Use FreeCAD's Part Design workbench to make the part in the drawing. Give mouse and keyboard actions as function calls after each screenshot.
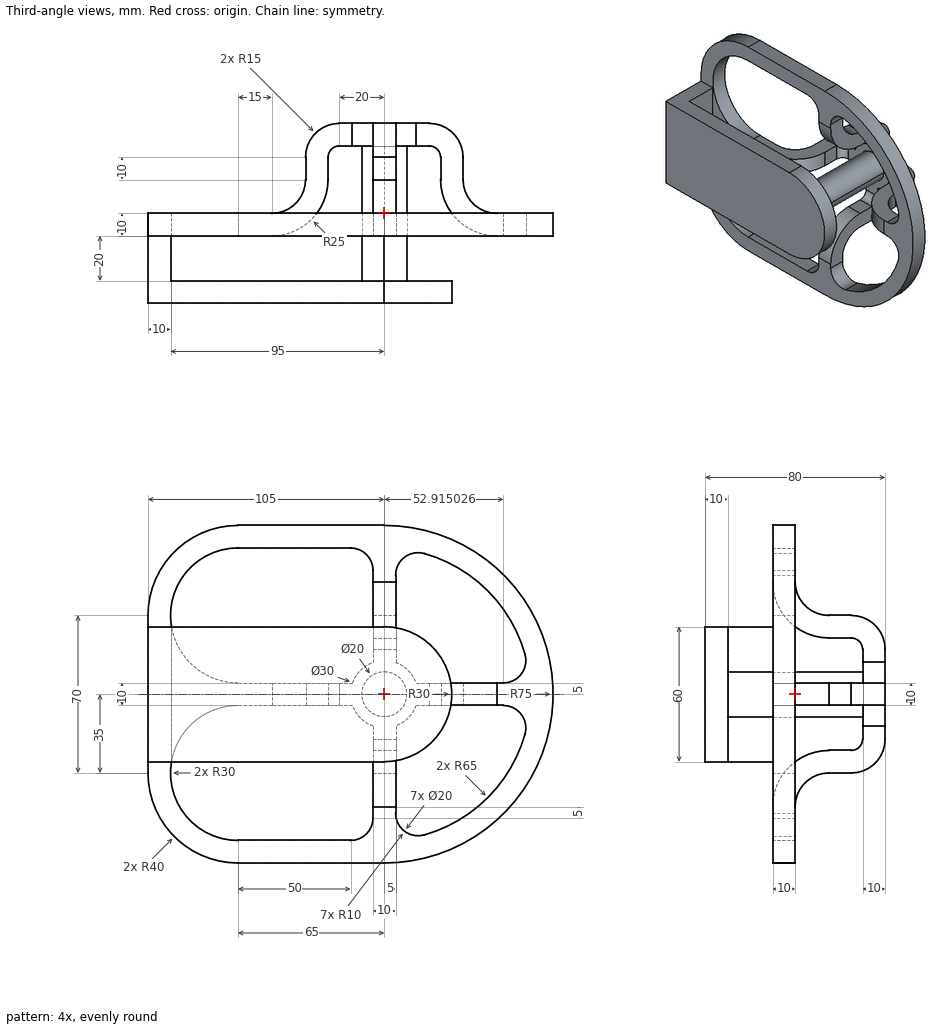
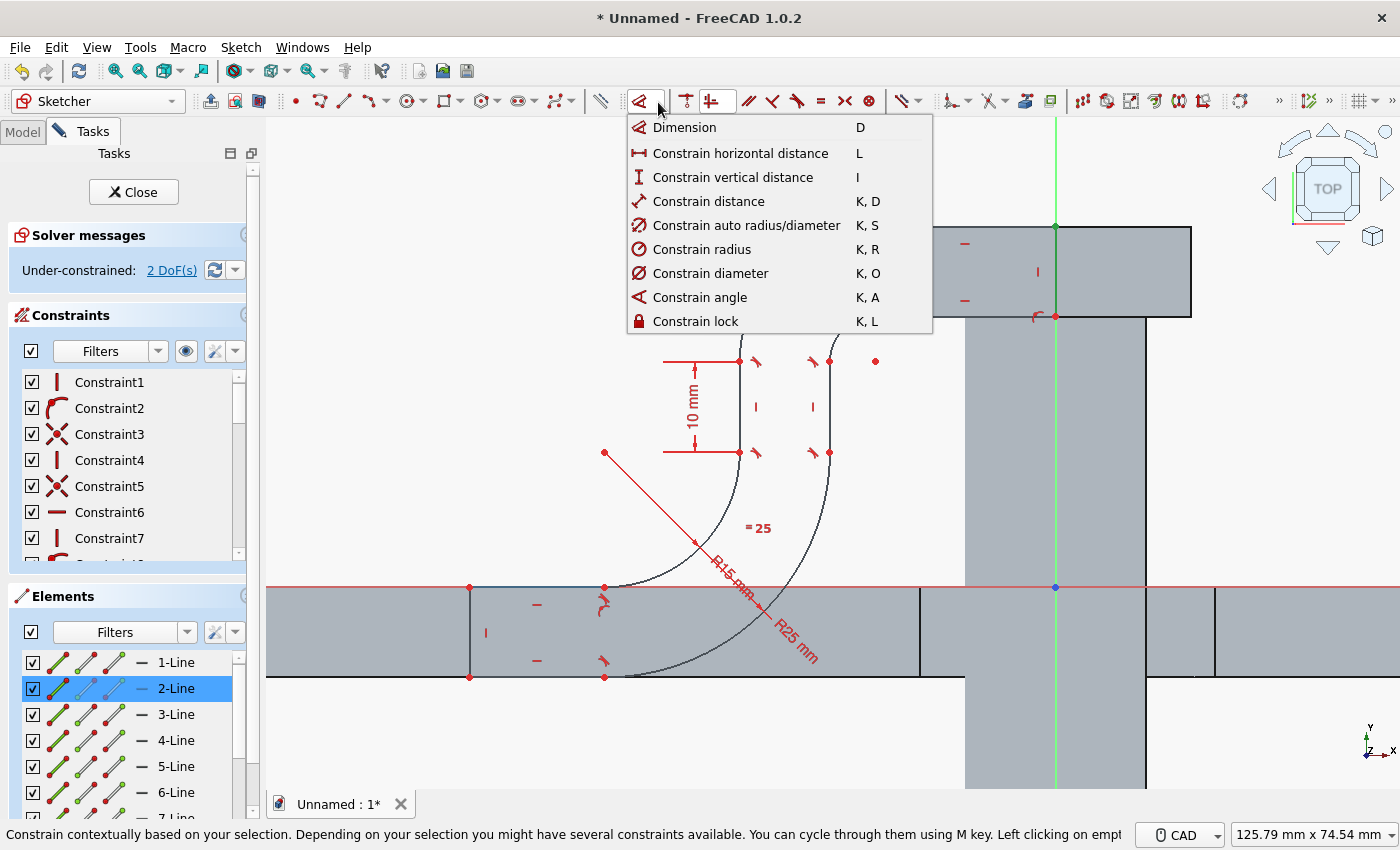
click(780, 153)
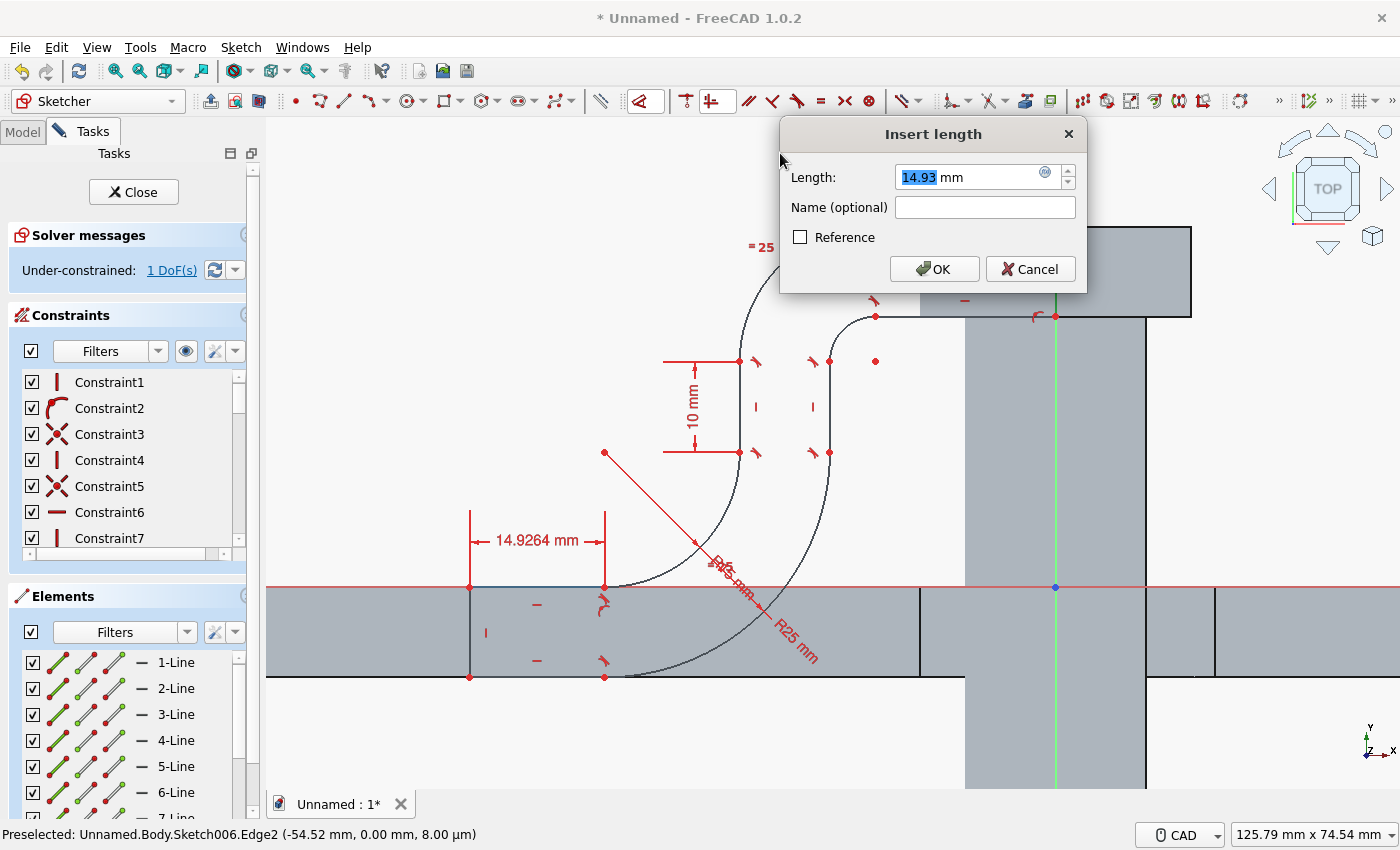
text(15)
key(Return)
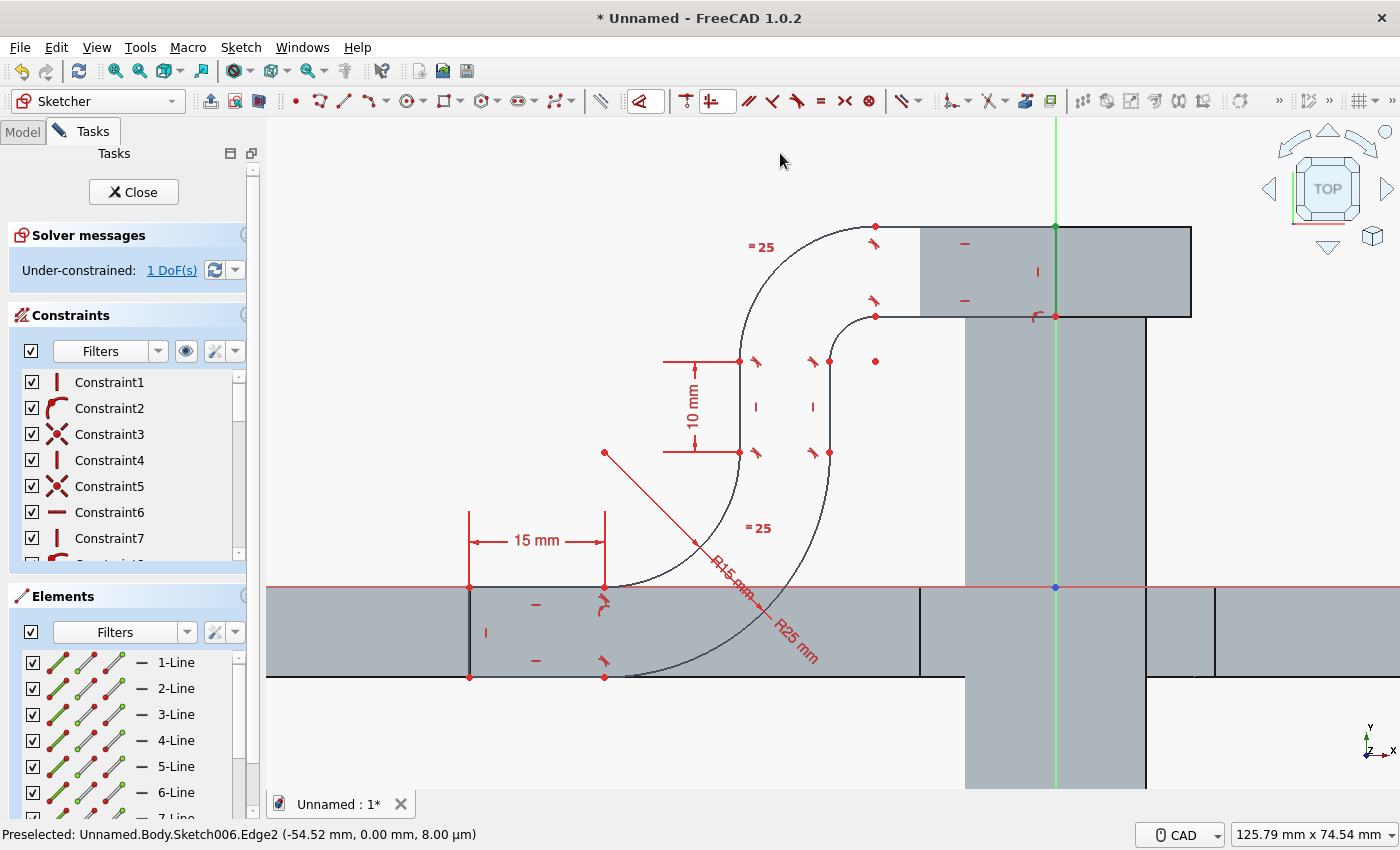
click(929, 317)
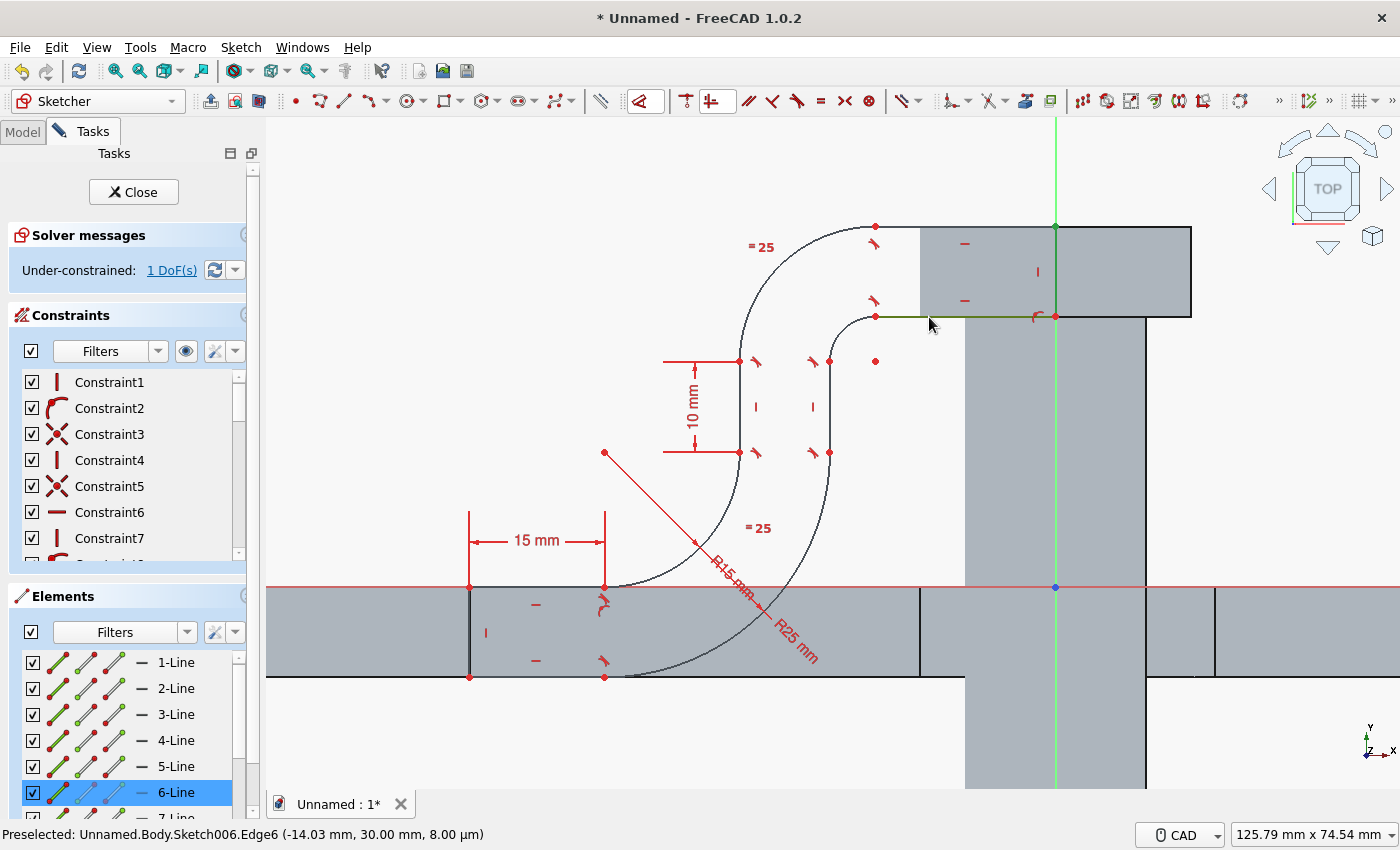
click(658, 102)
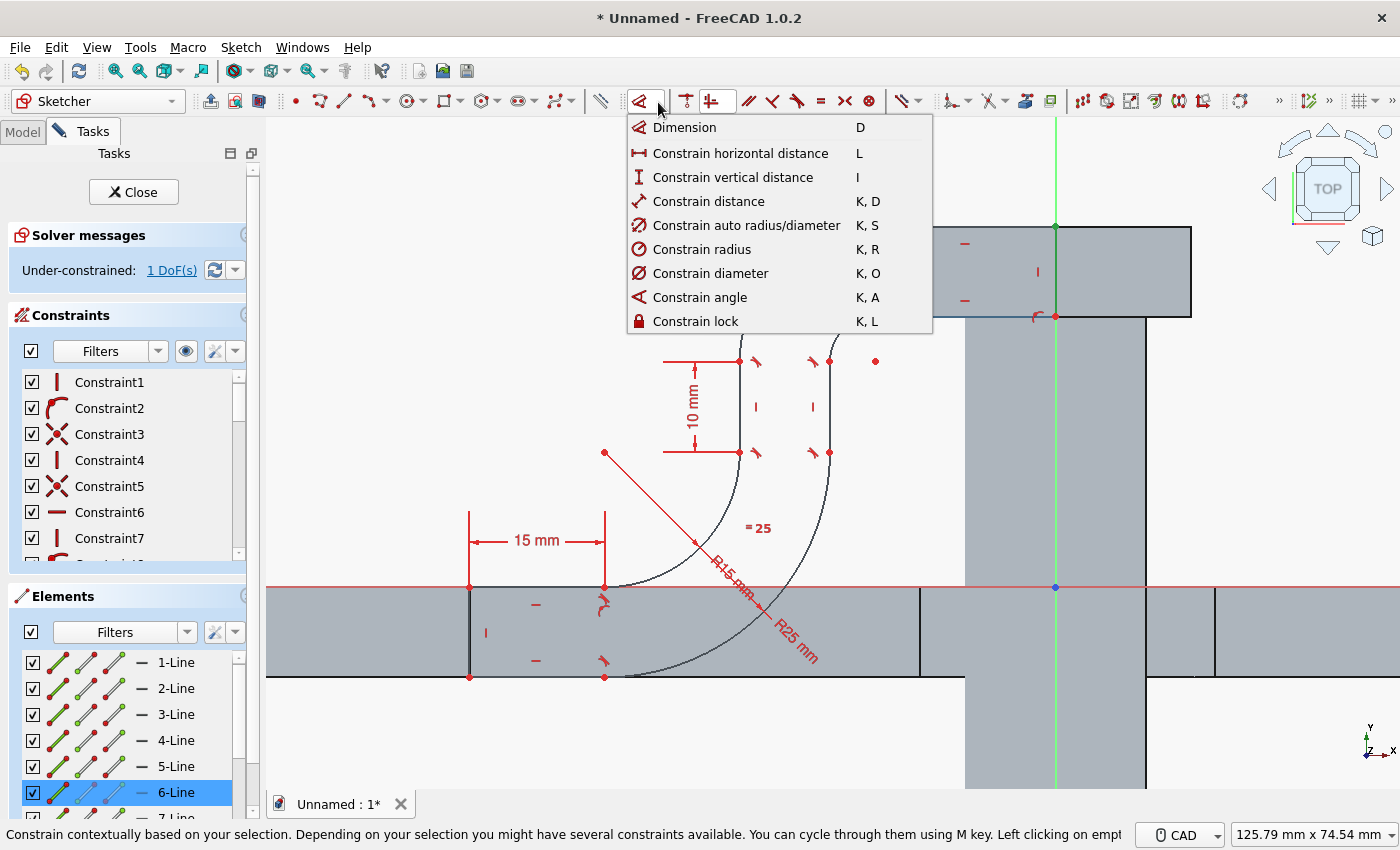
click(780, 153)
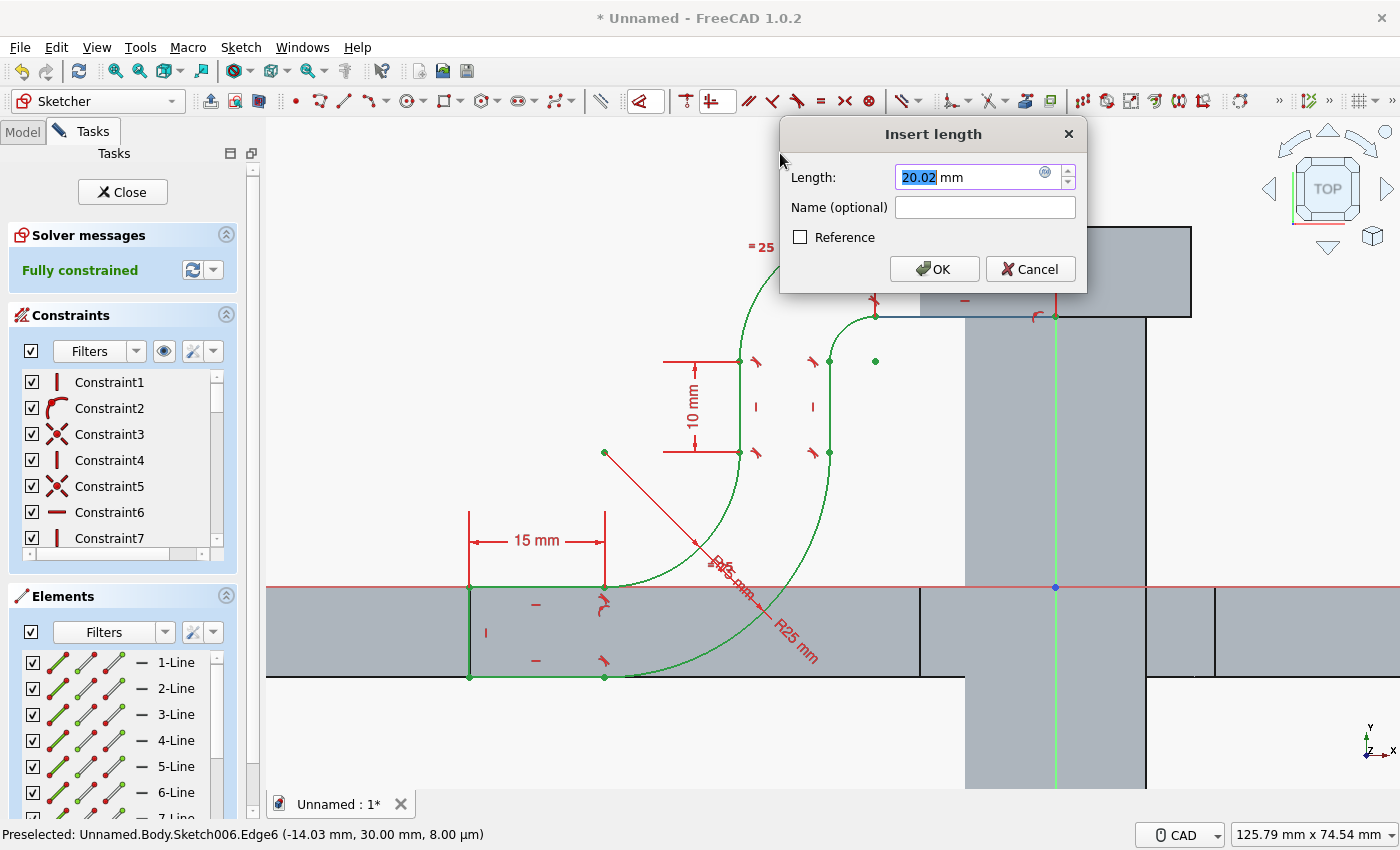
text(20)
key(Return)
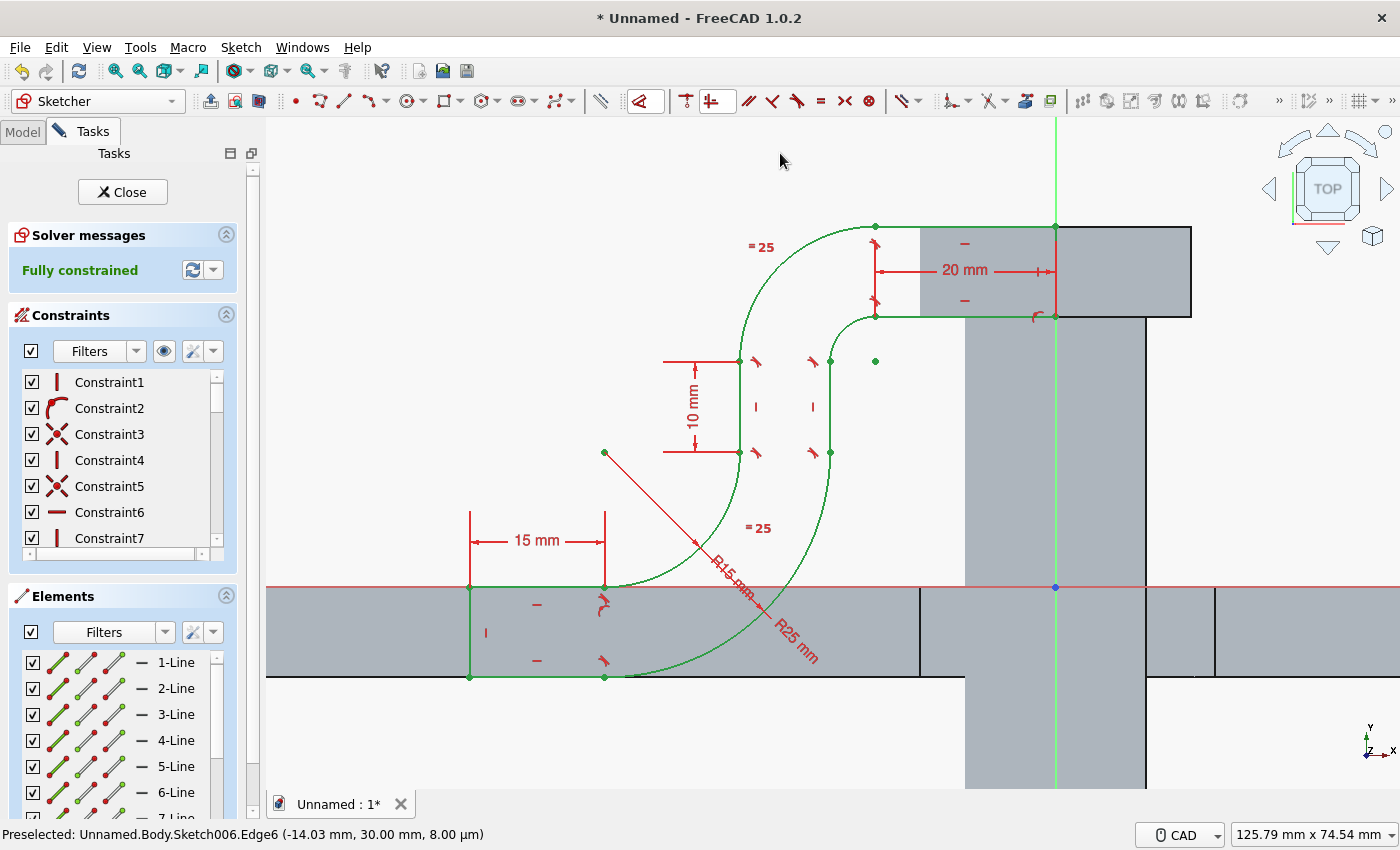
click(123, 192)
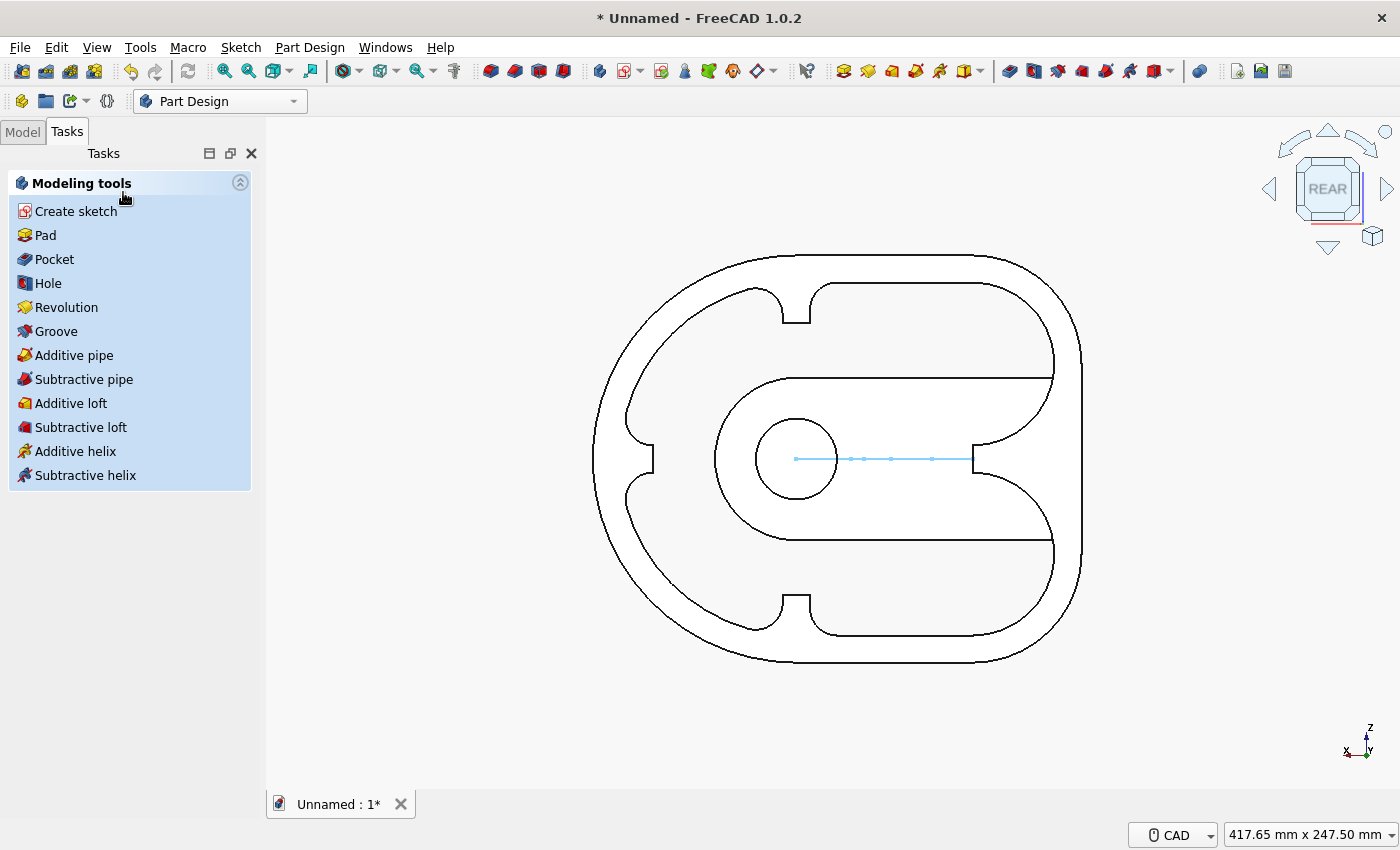
click(844, 72)